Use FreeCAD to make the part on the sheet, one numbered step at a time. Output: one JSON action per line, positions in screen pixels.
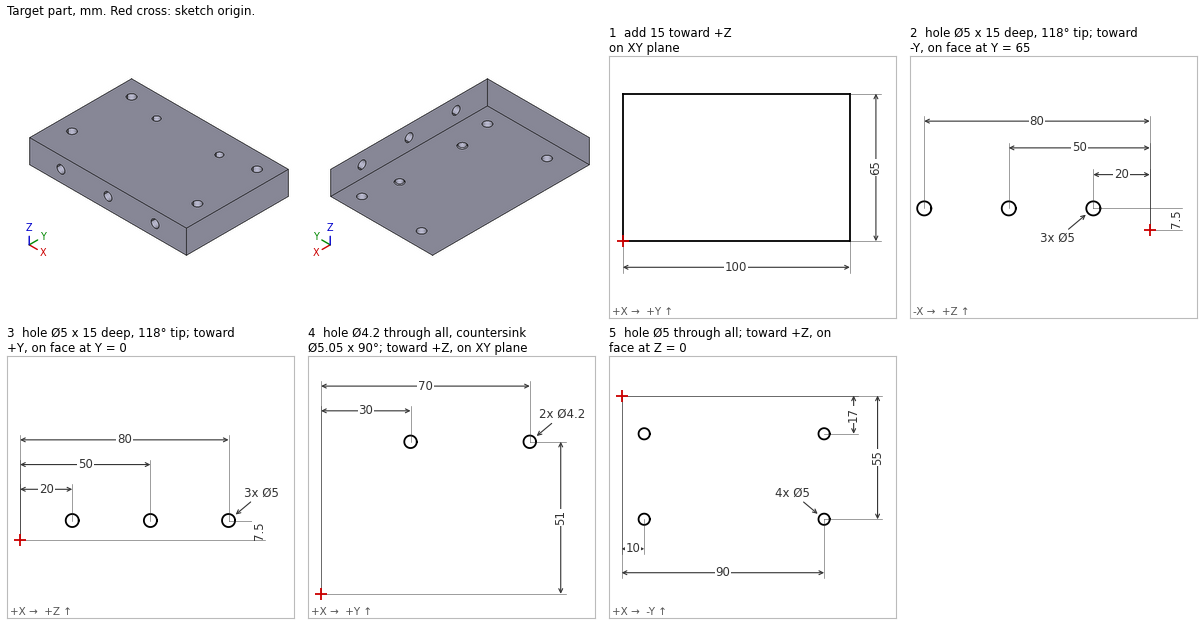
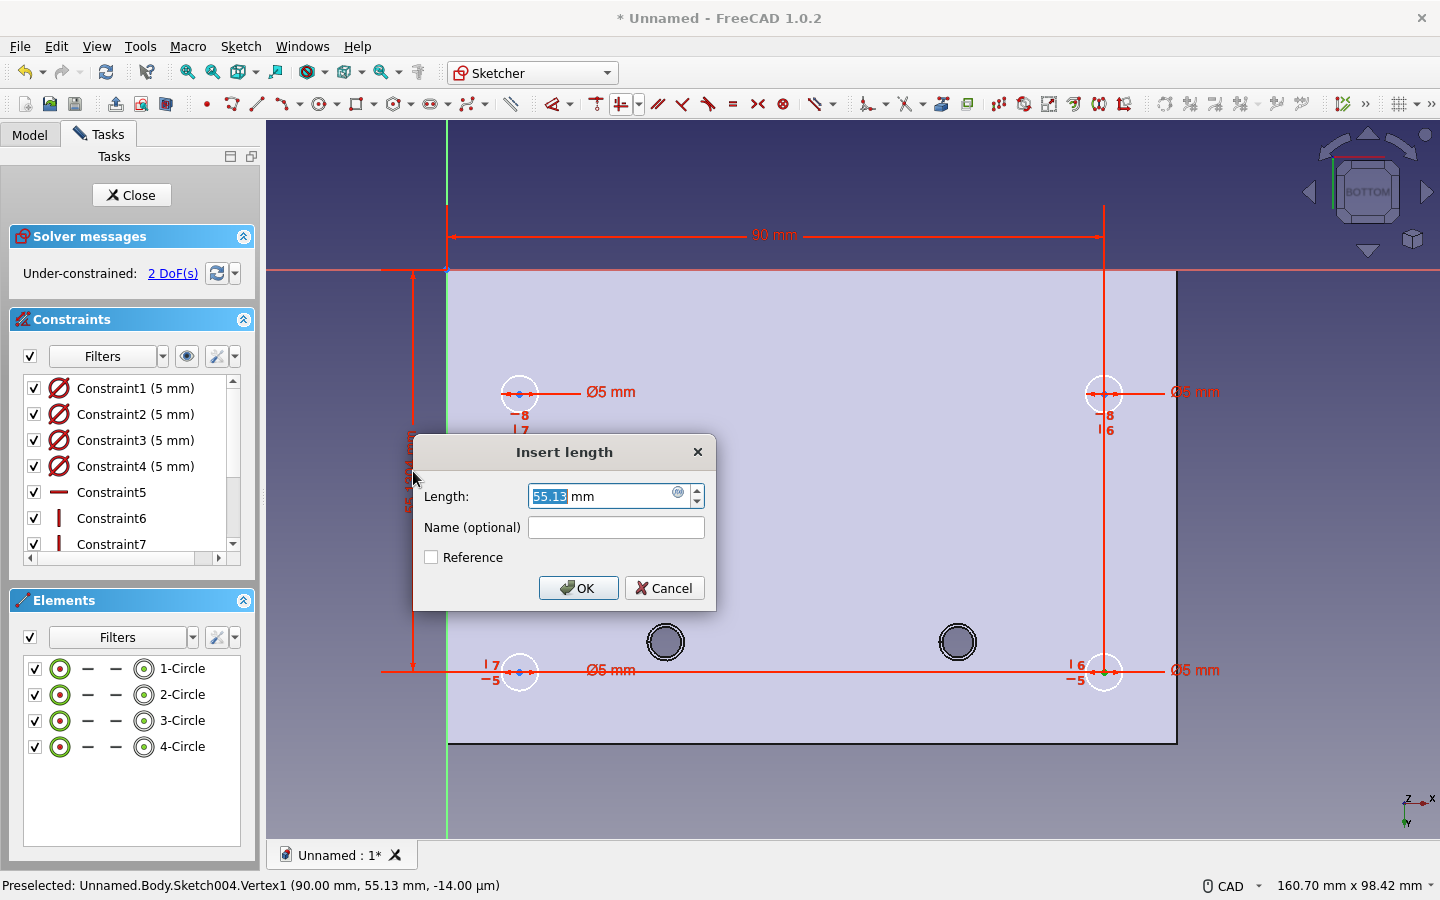
{"action": "type", "text": "55"}
{"action": "key", "text": "Return"}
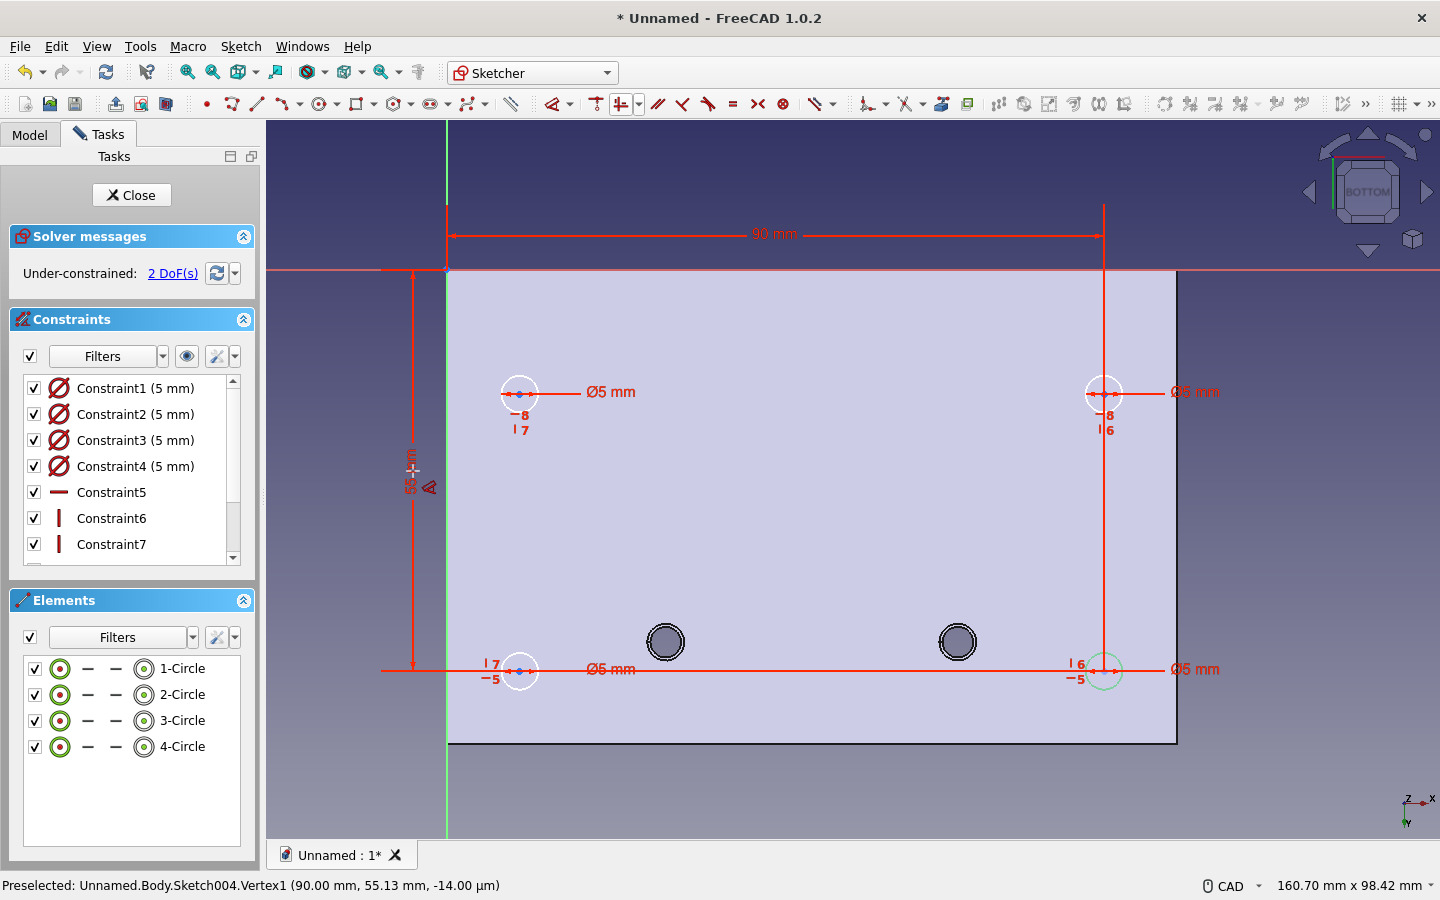
{"action": "left_click", "coordinate": [520, 671]}
{"action": "left_click", "coordinate": [483, 236]}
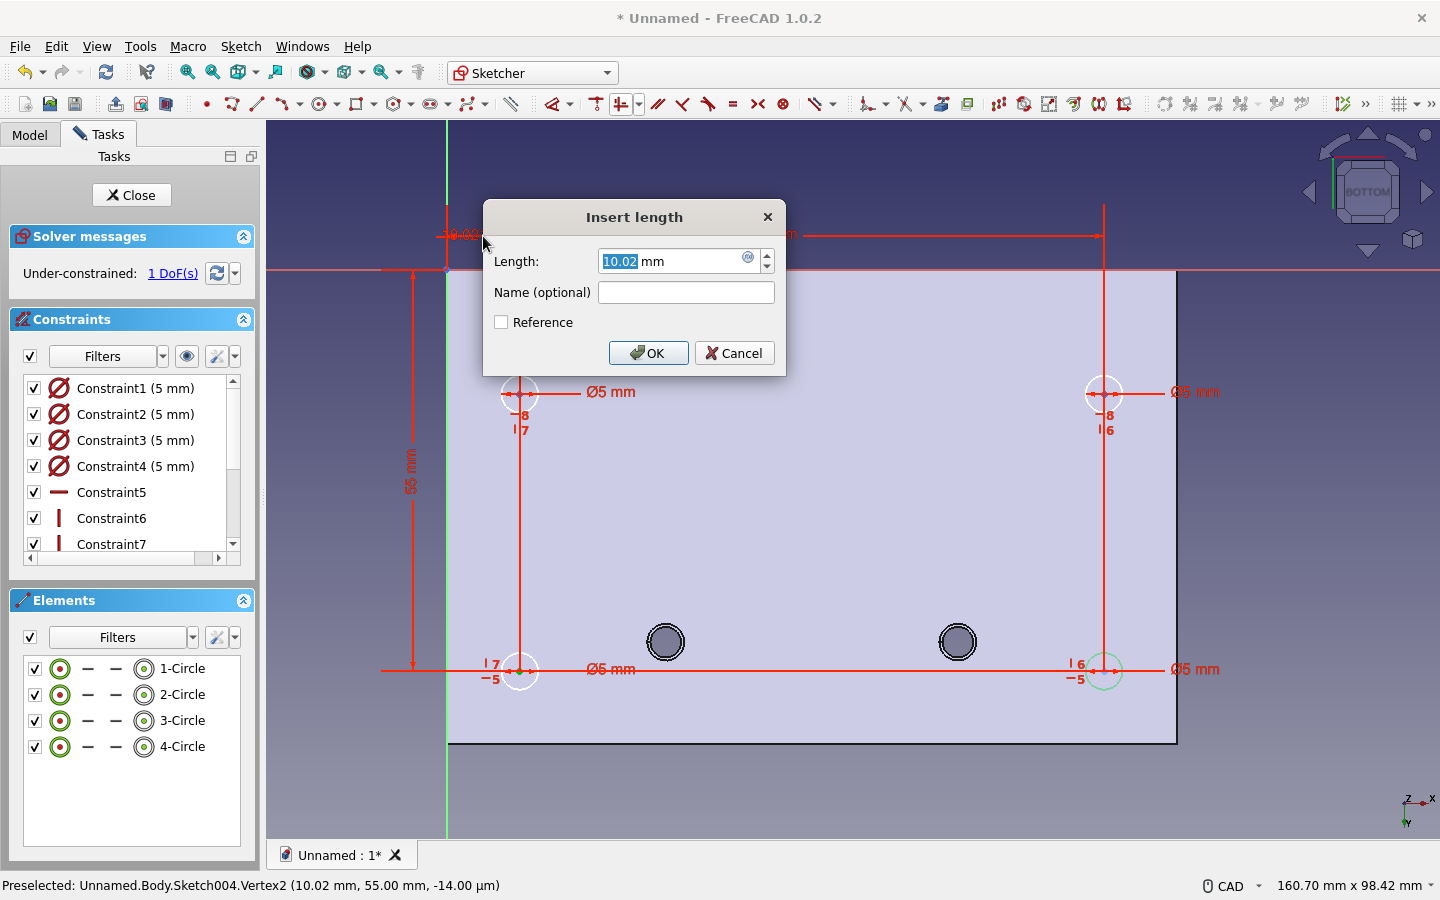
{"action": "type", "text": "10"}
{"action": "key", "text": "Return"}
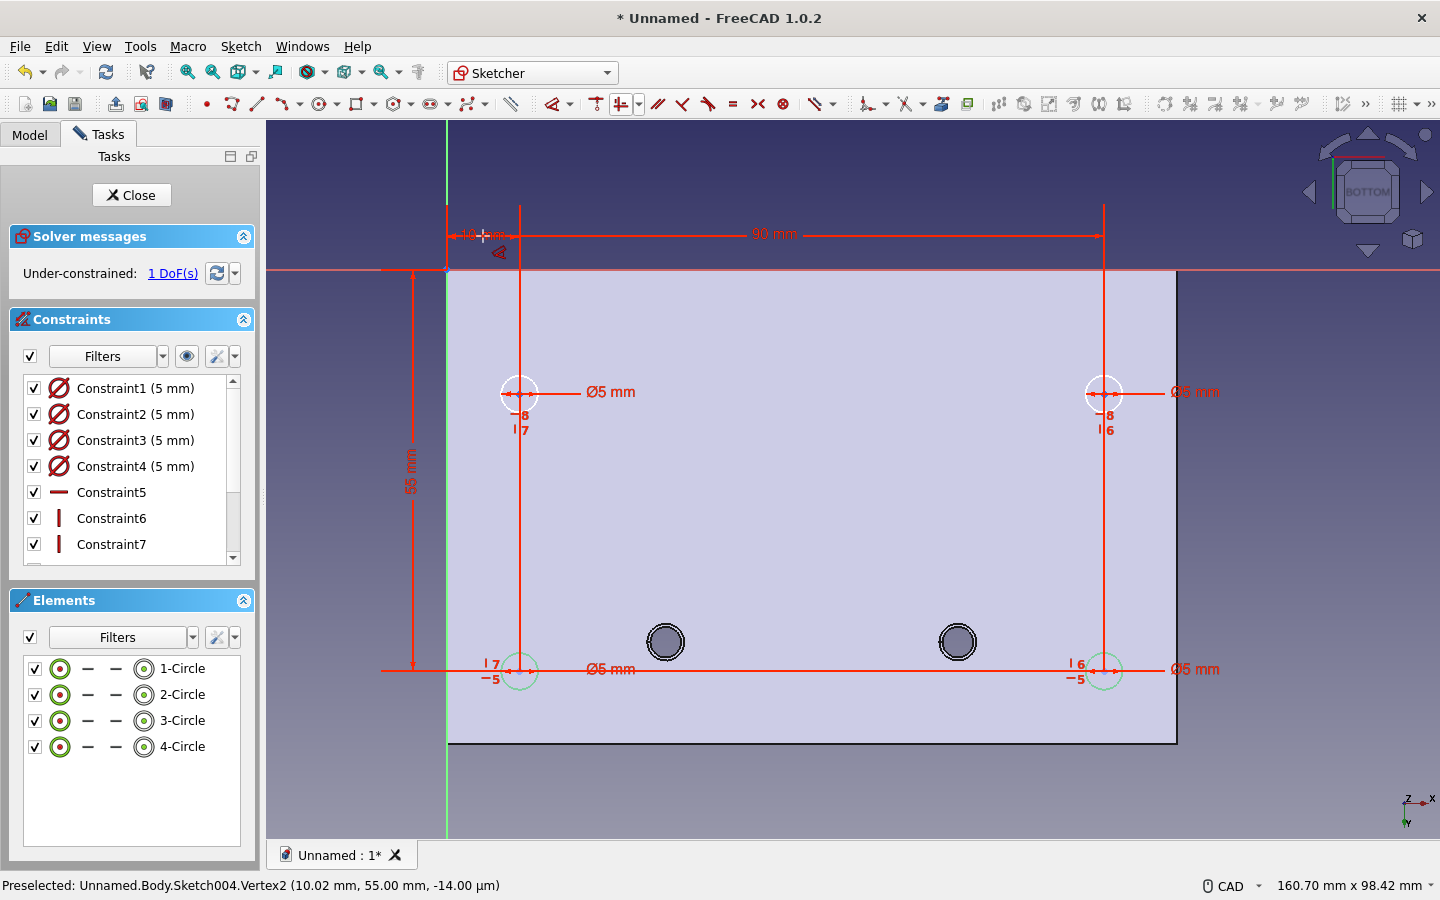
{"action": "left_click", "coordinate": [1104, 394]}
{"action": "left_click", "coordinate": [413, 332]}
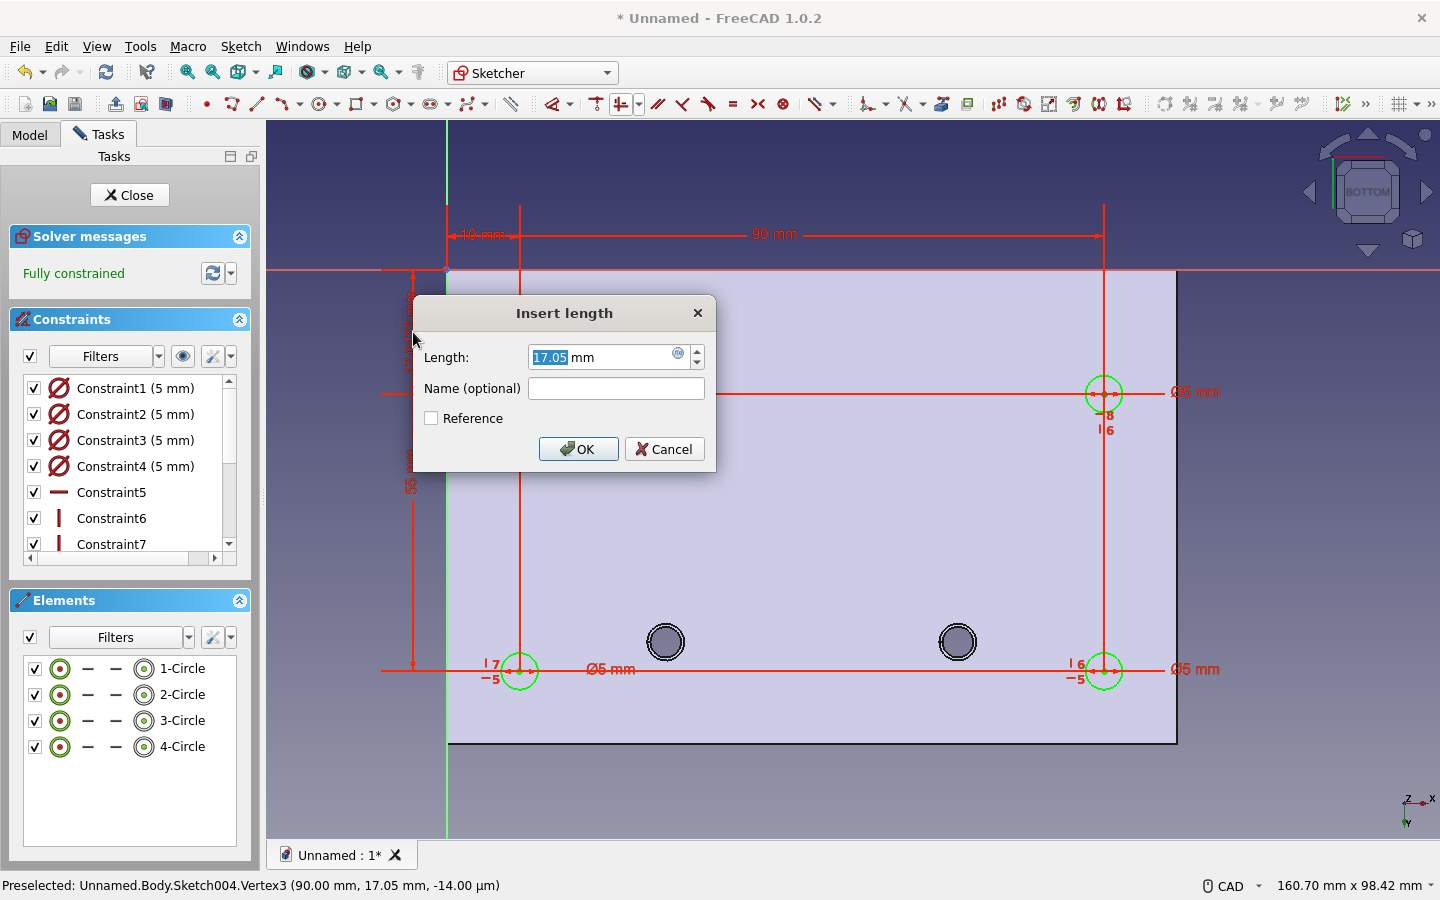
{"action": "type", "text": "17"}
{"action": "key", "text": "Return"}
{"action": "key", "text": "Escape"}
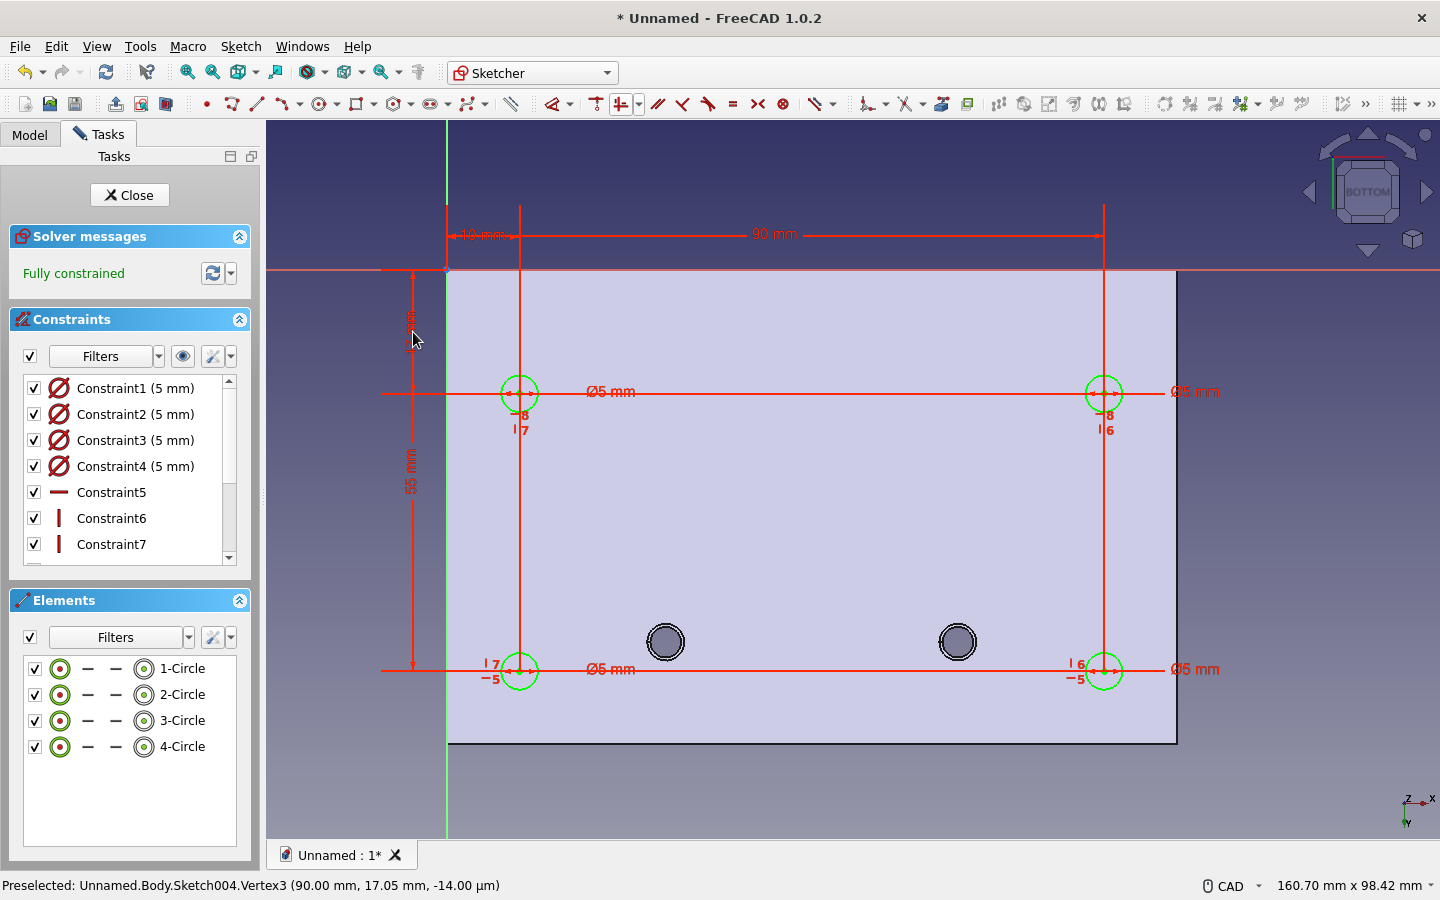
{"action": "left_click", "coordinate": [130, 195]}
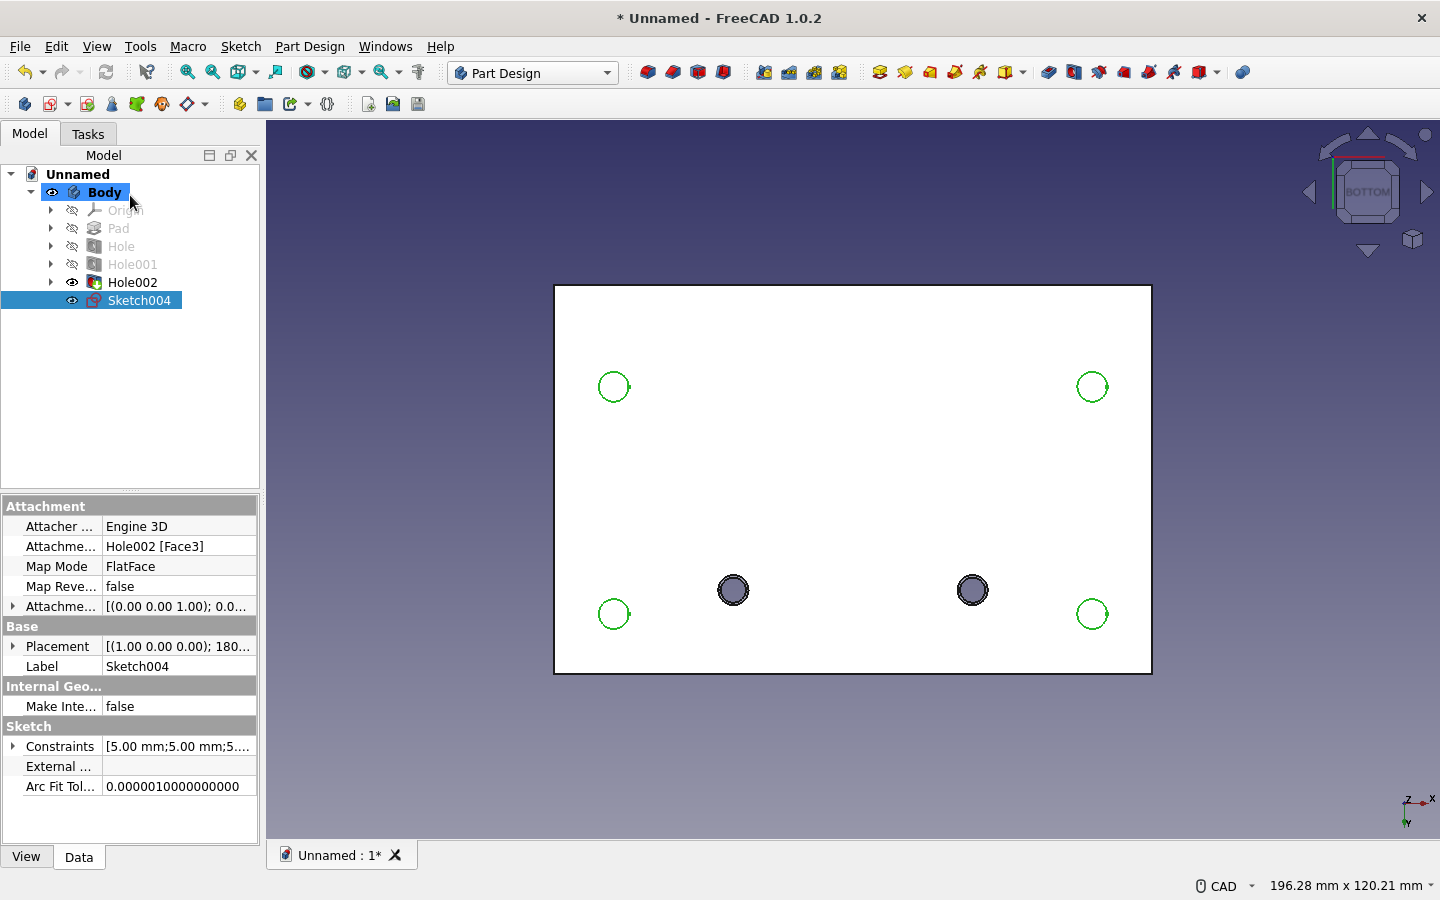
{"action": "left_click", "coordinate": [1074, 72]}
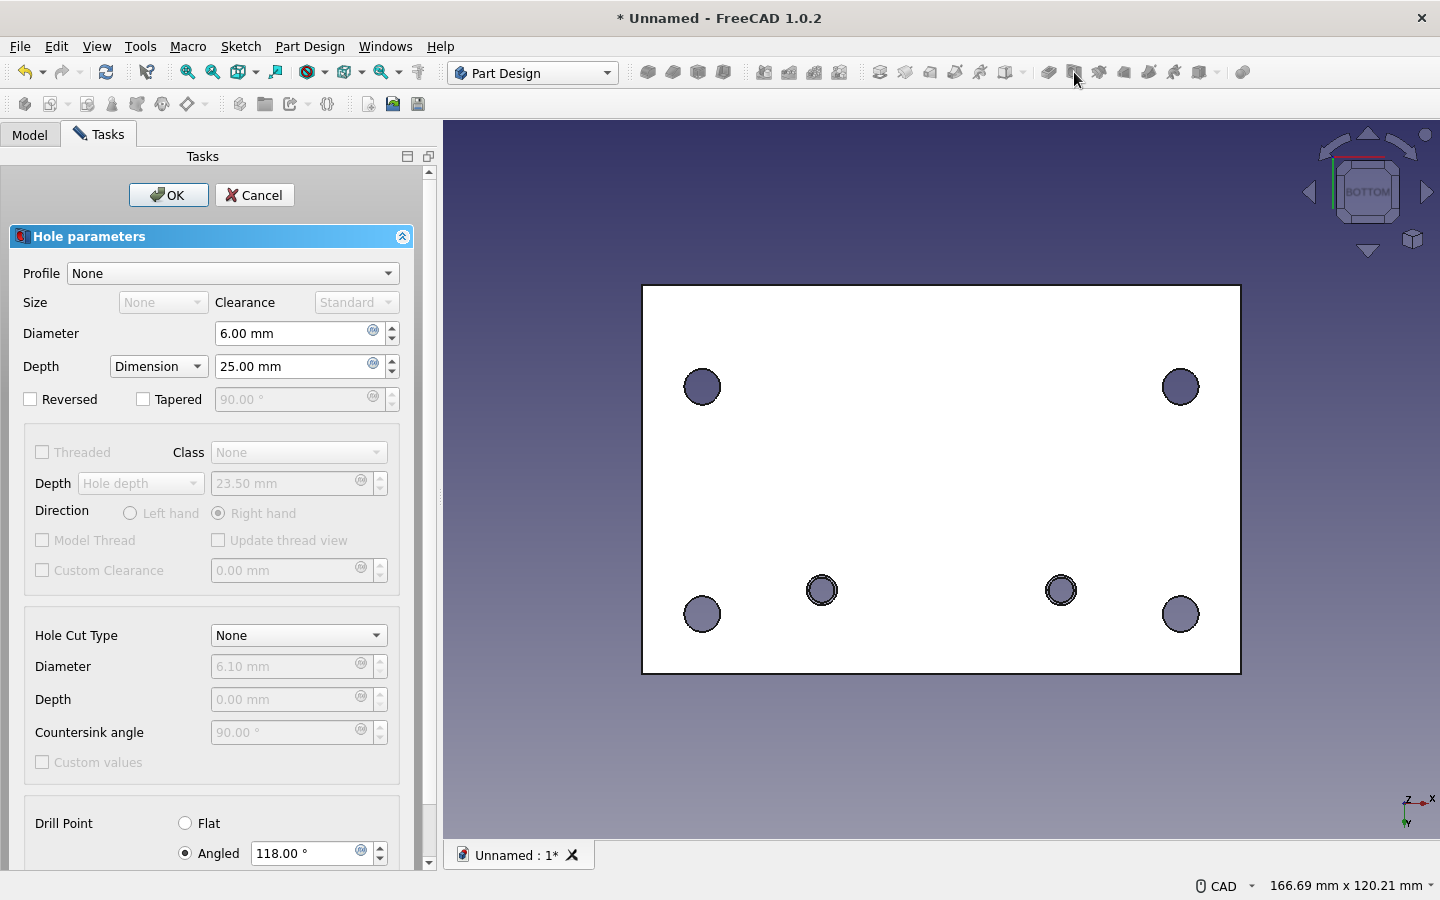
{"action": "triple_click", "coordinate": [300, 334]}